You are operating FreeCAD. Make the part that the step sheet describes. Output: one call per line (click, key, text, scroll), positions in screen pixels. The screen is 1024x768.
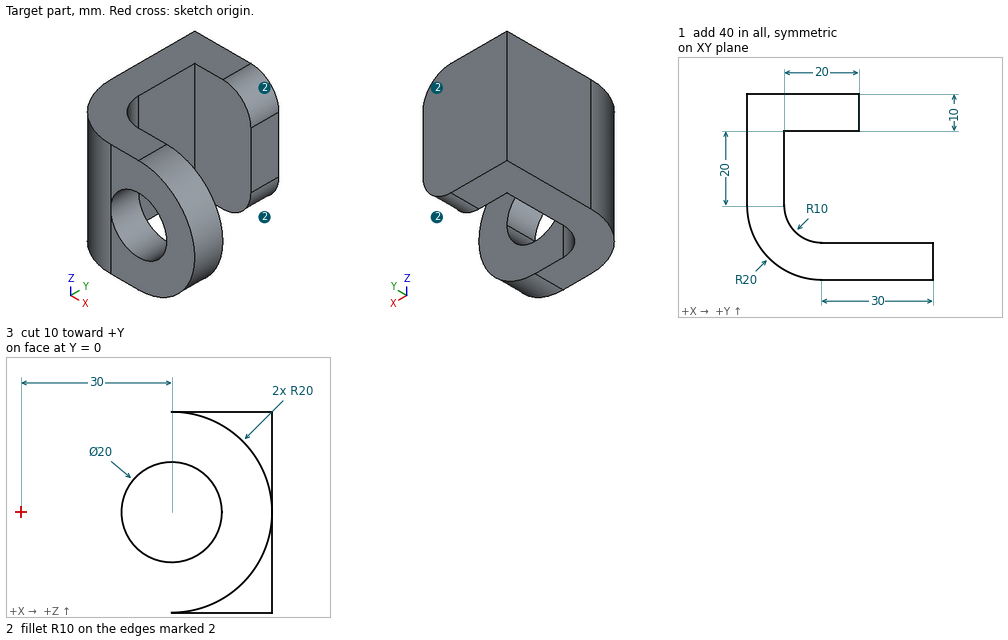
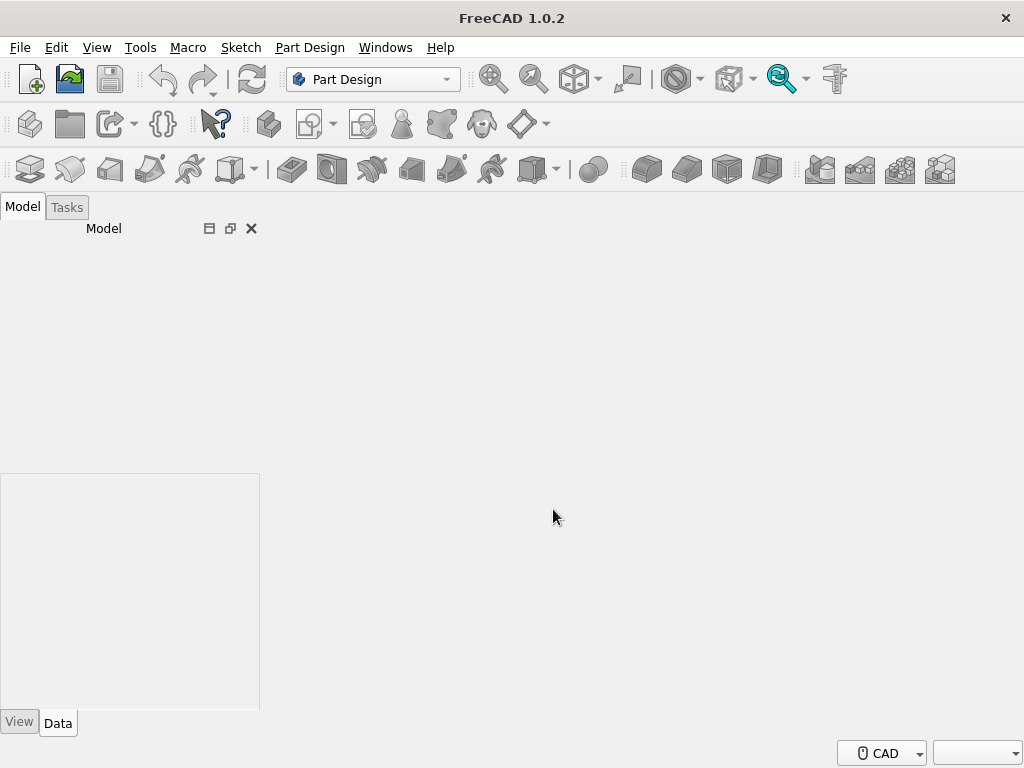
click(30, 80)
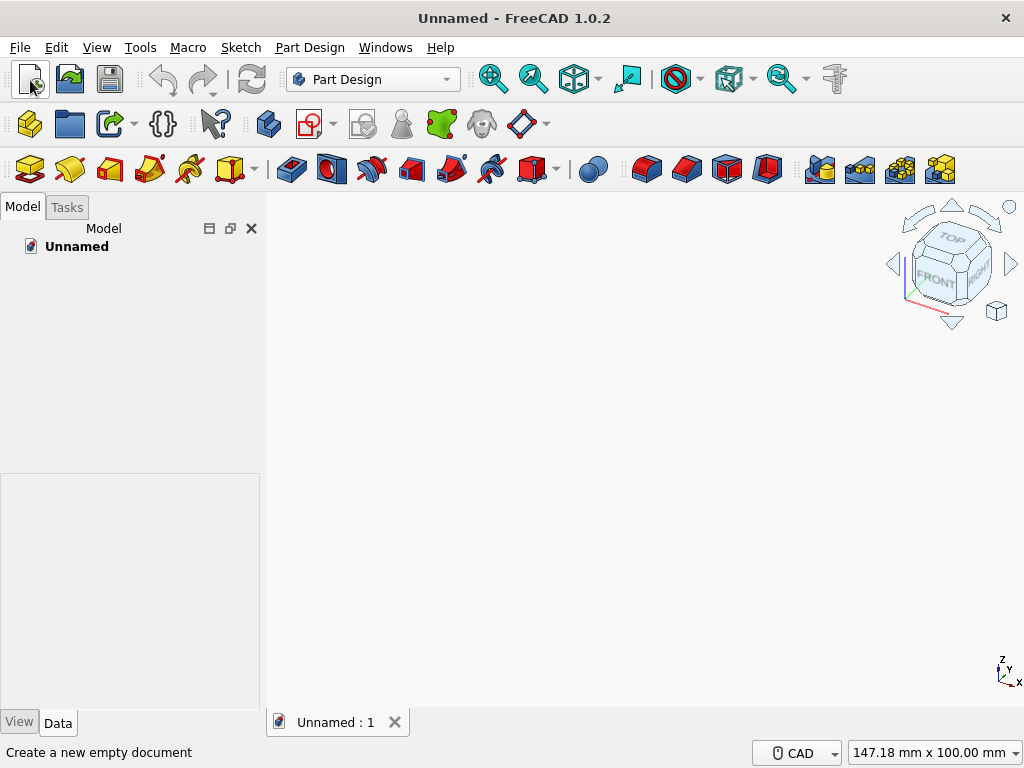
click(310, 124)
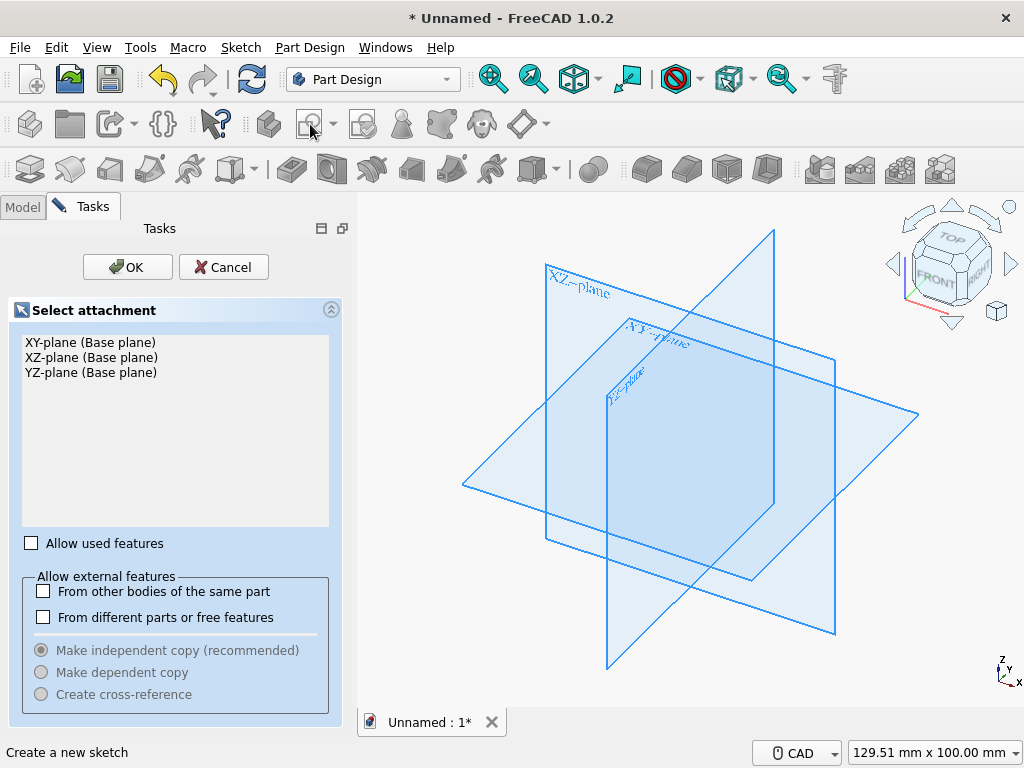
click(82, 342)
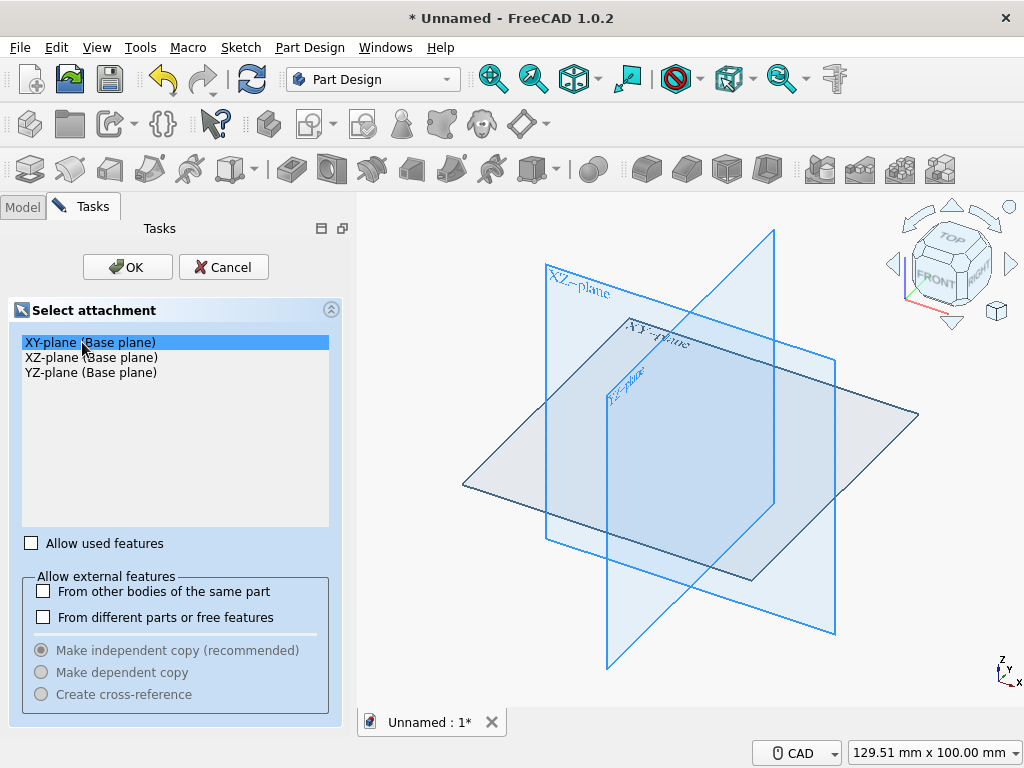
click(128, 267)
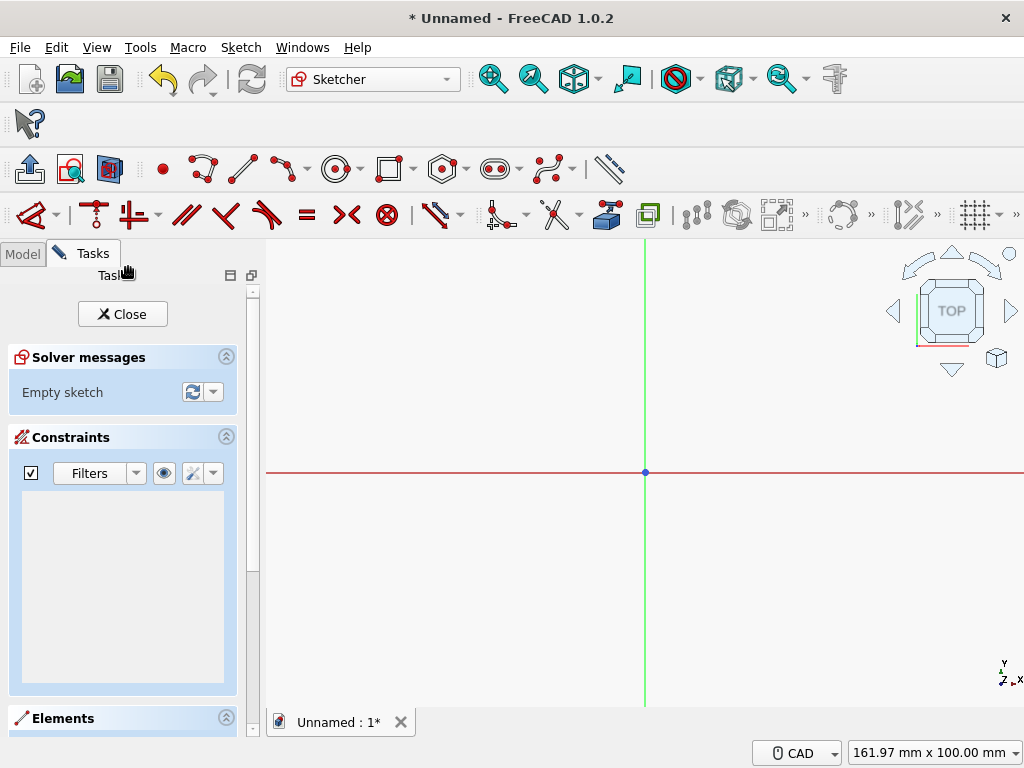
scroll(294, 679, down, 1)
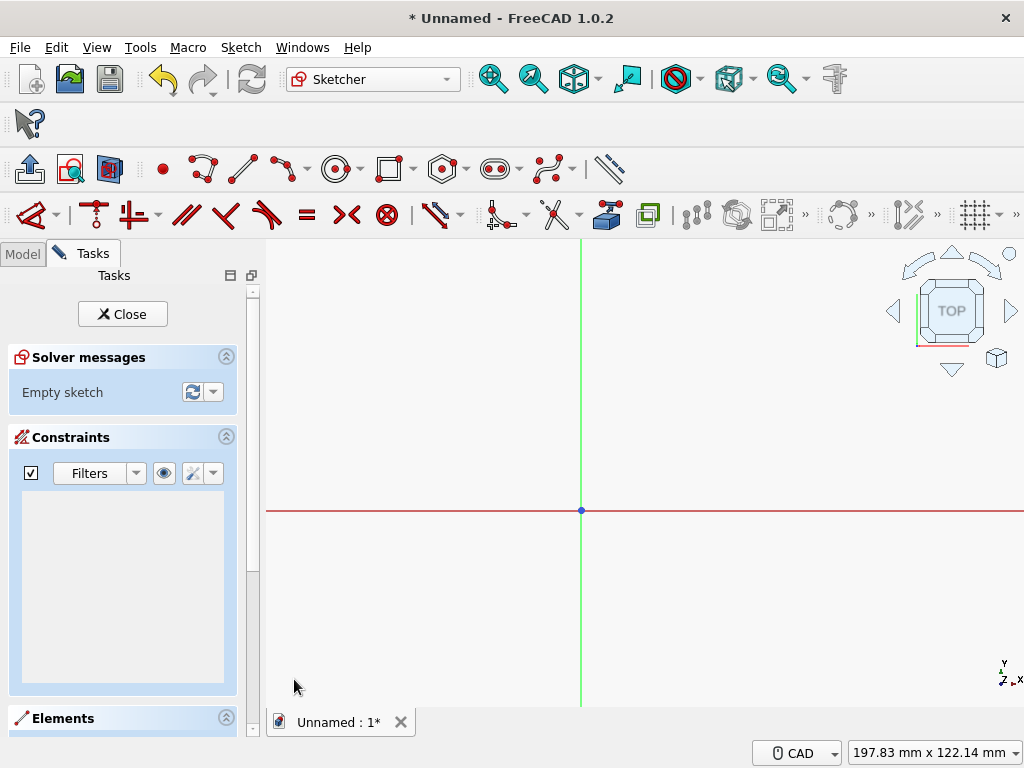
scroll(859, 296, up, 2)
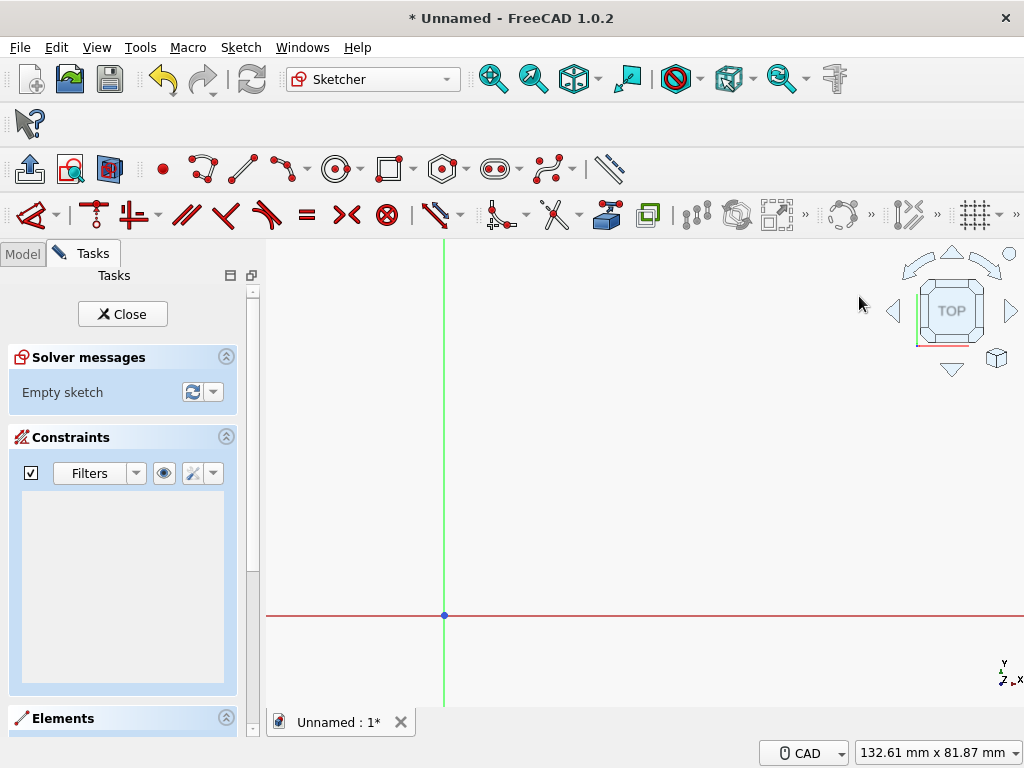
click(204, 170)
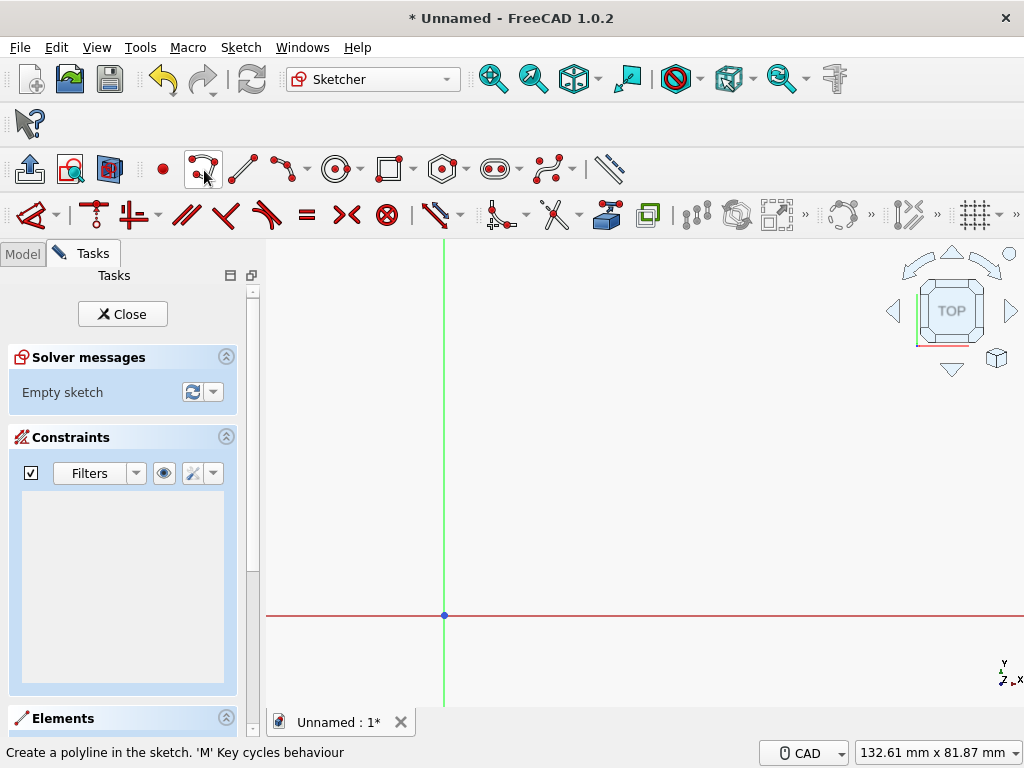
click(559, 616)
click(730, 607)
click(730, 559)
click(559, 559)
right_click(559, 559)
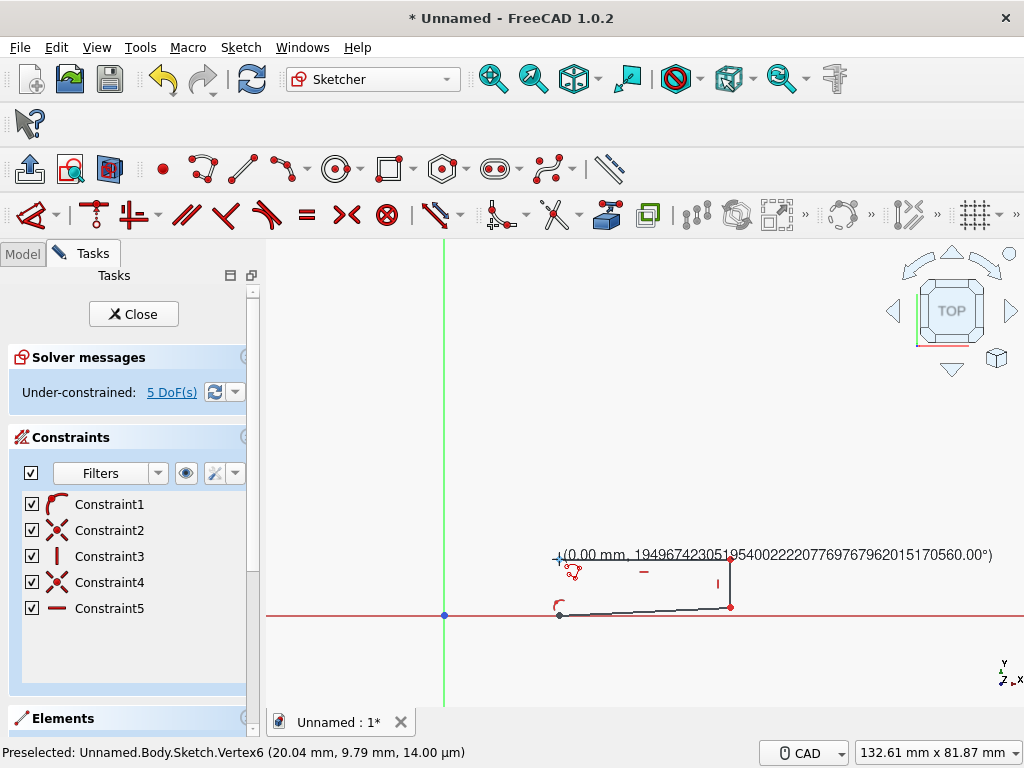
click(502, 502)
click(502, 387)
click(616, 387)
click(616, 330)
click(444, 330)
click(453, 502)
right_click(453, 502)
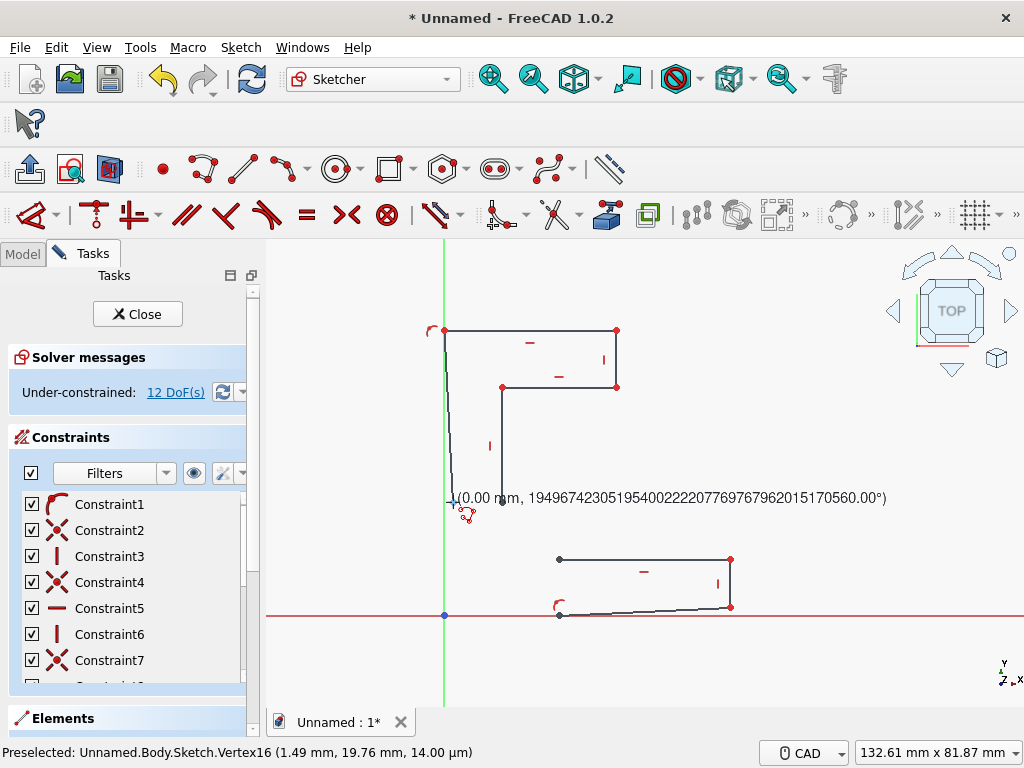
click(284, 170)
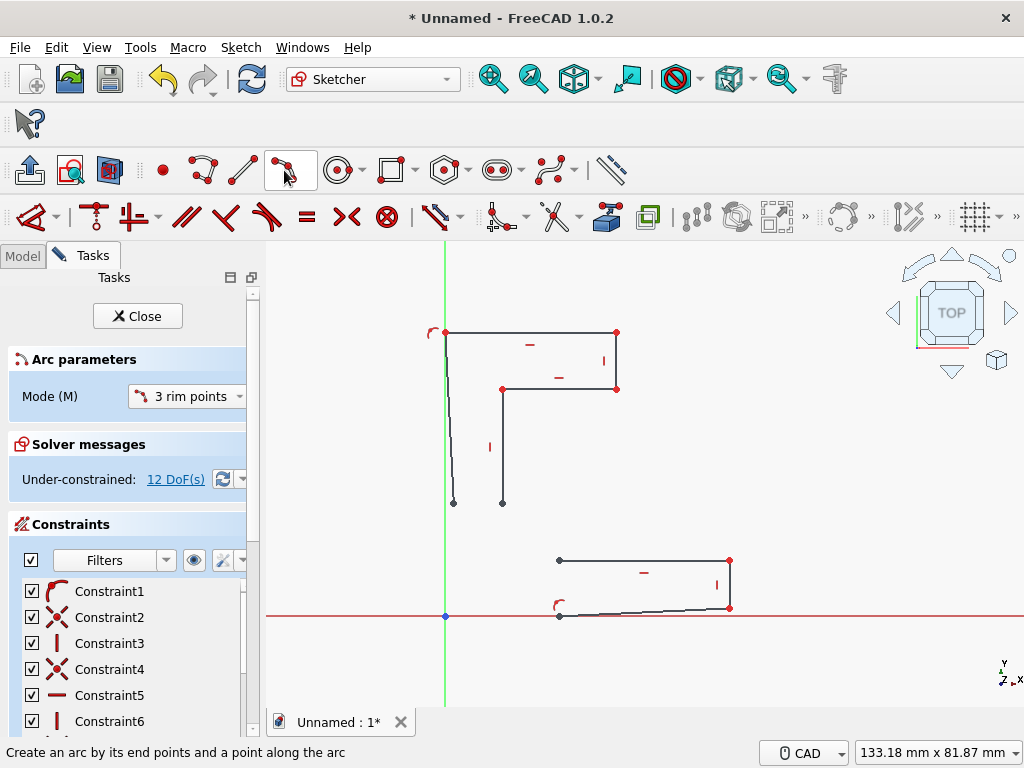
click(559, 561)
click(503, 504)
click(519, 543)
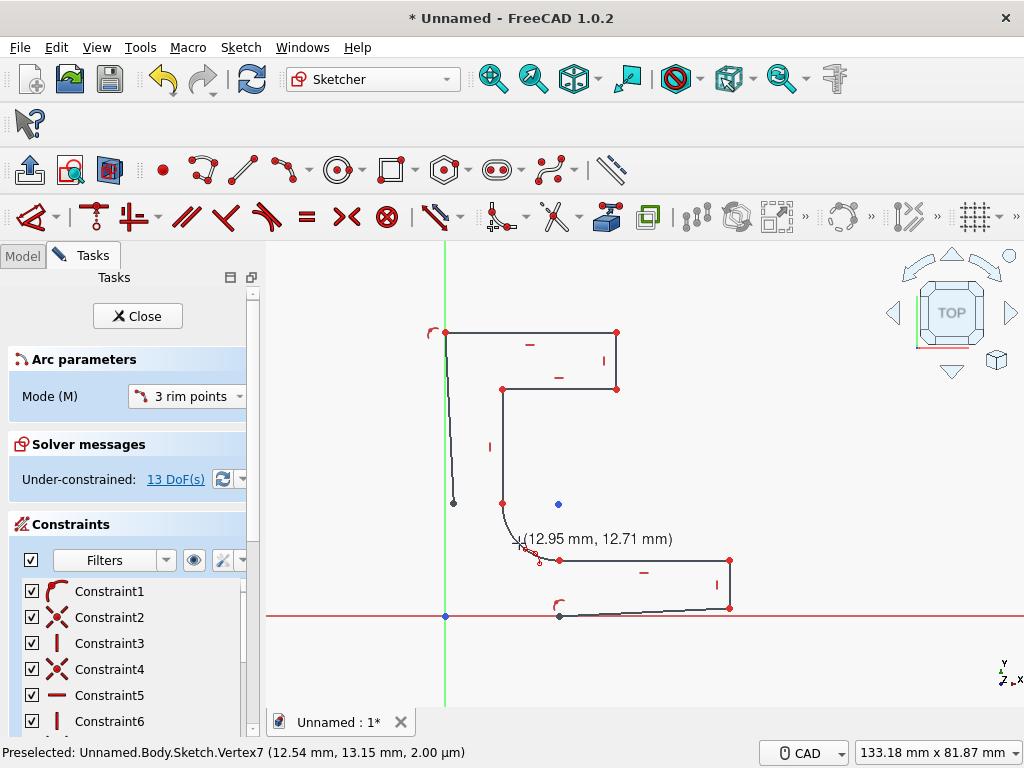
click(454, 504)
click(559, 616)
click(479, 583)
key(Escape)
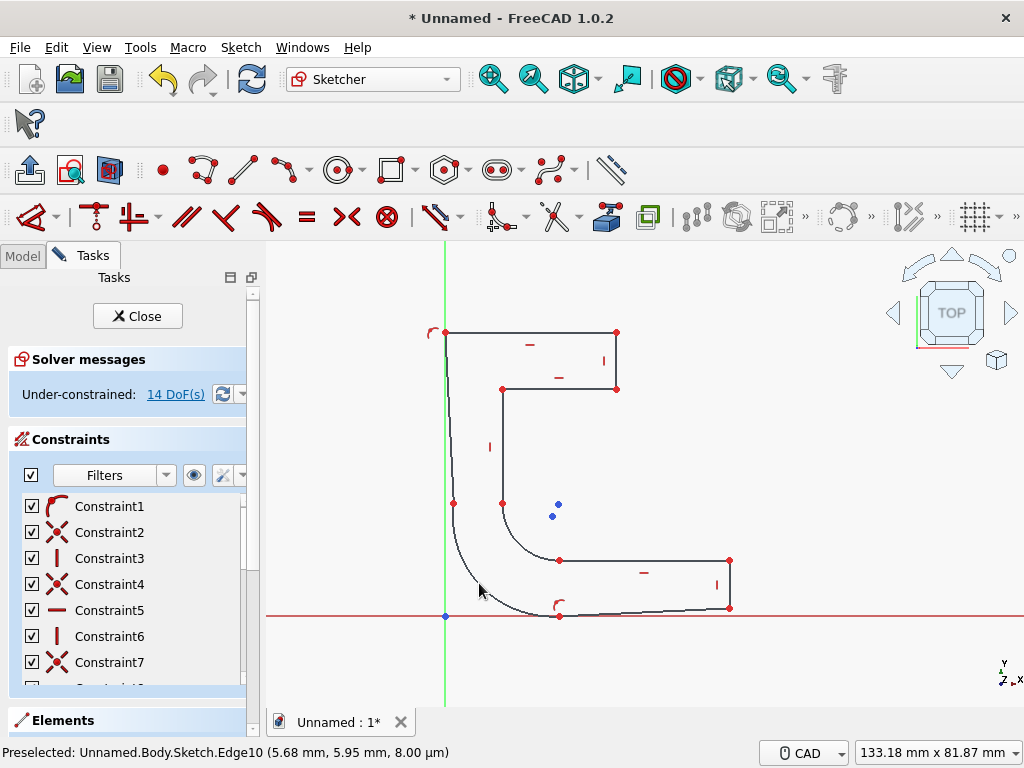
click(610, 614)